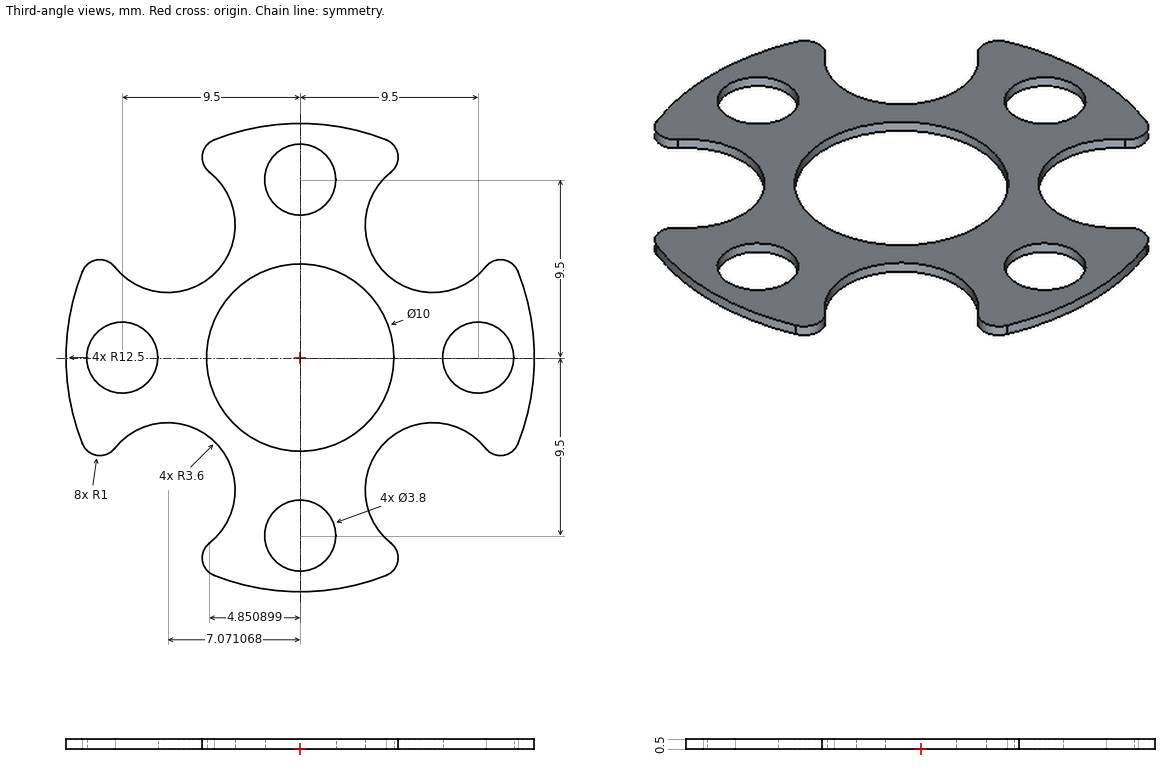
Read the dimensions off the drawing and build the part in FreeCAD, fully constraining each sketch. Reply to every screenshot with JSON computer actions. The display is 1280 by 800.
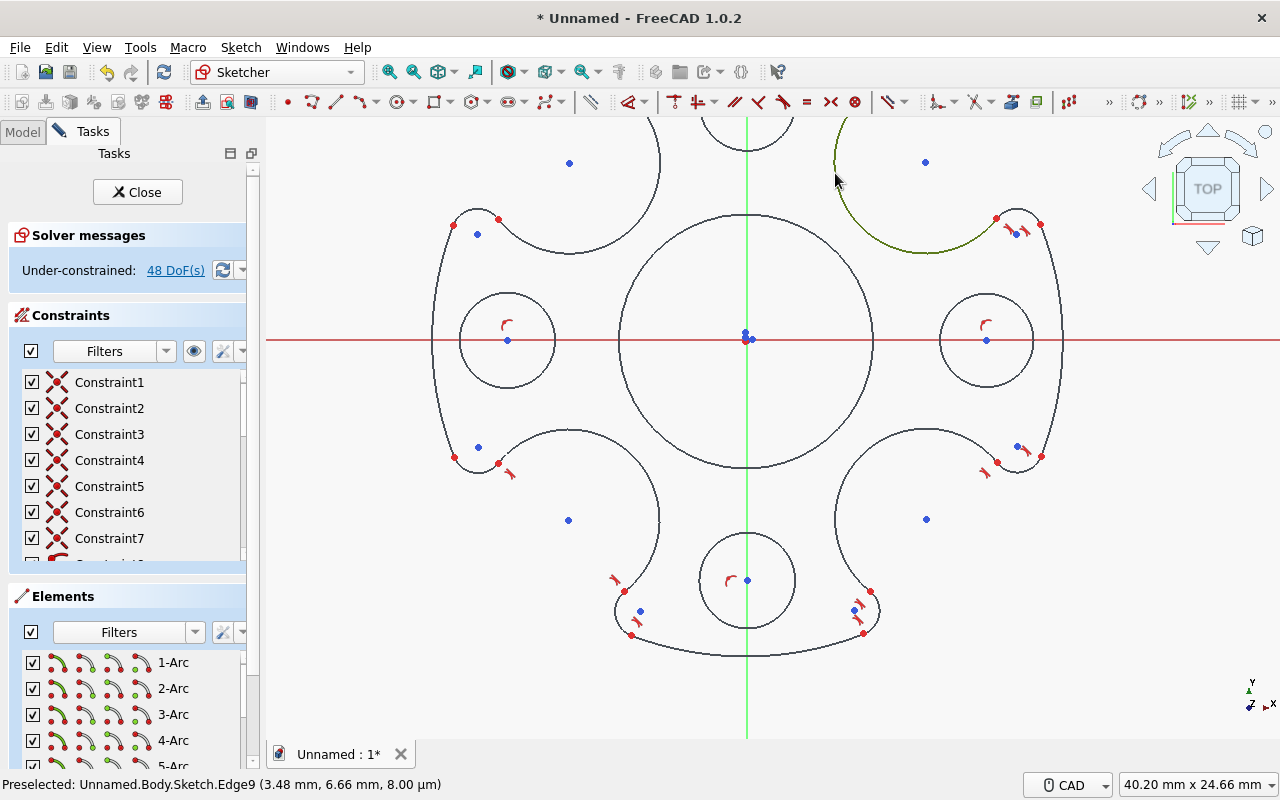
{"action": "scroll", "coordinate": [618, 606], "scroll_direction": "down", "scroll_amount": 2}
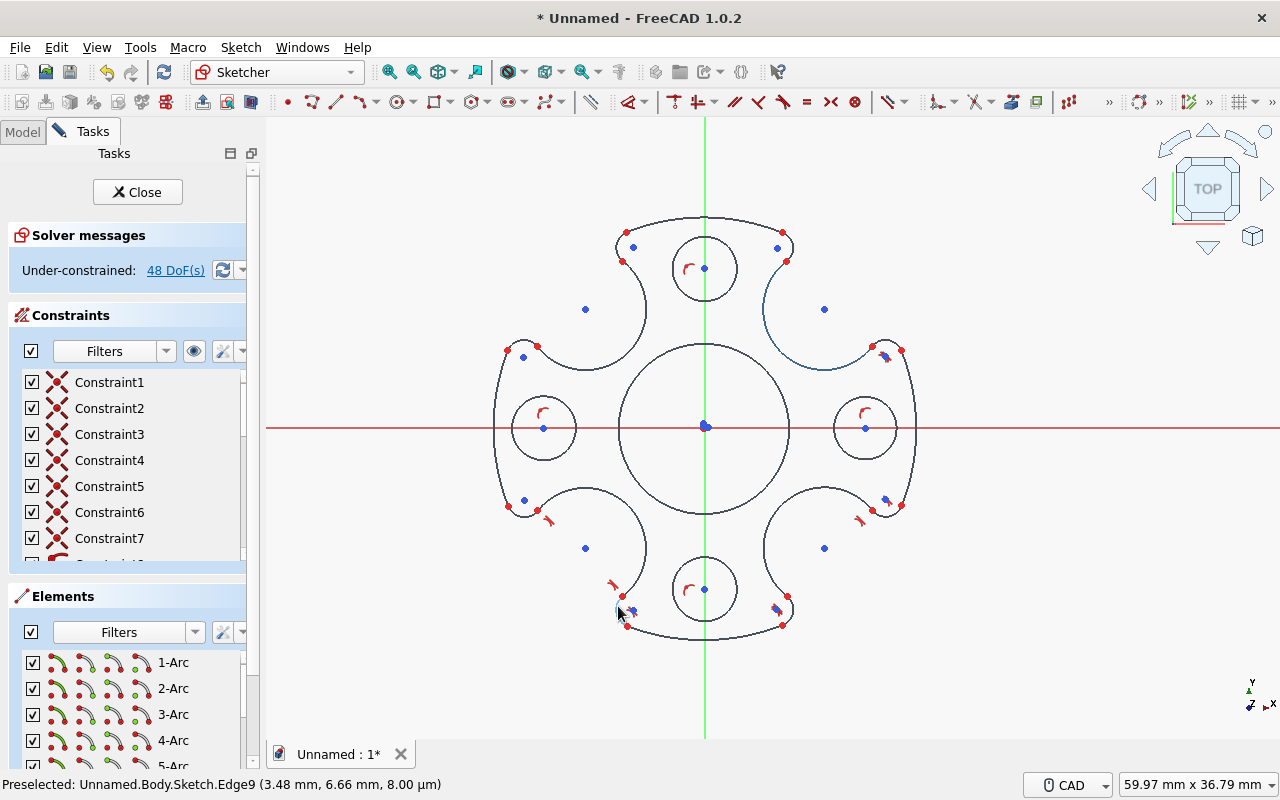
{"action": "scroll", "coordinate": [793, 253], "scroll_direction": "up", "scroll_amount": 2}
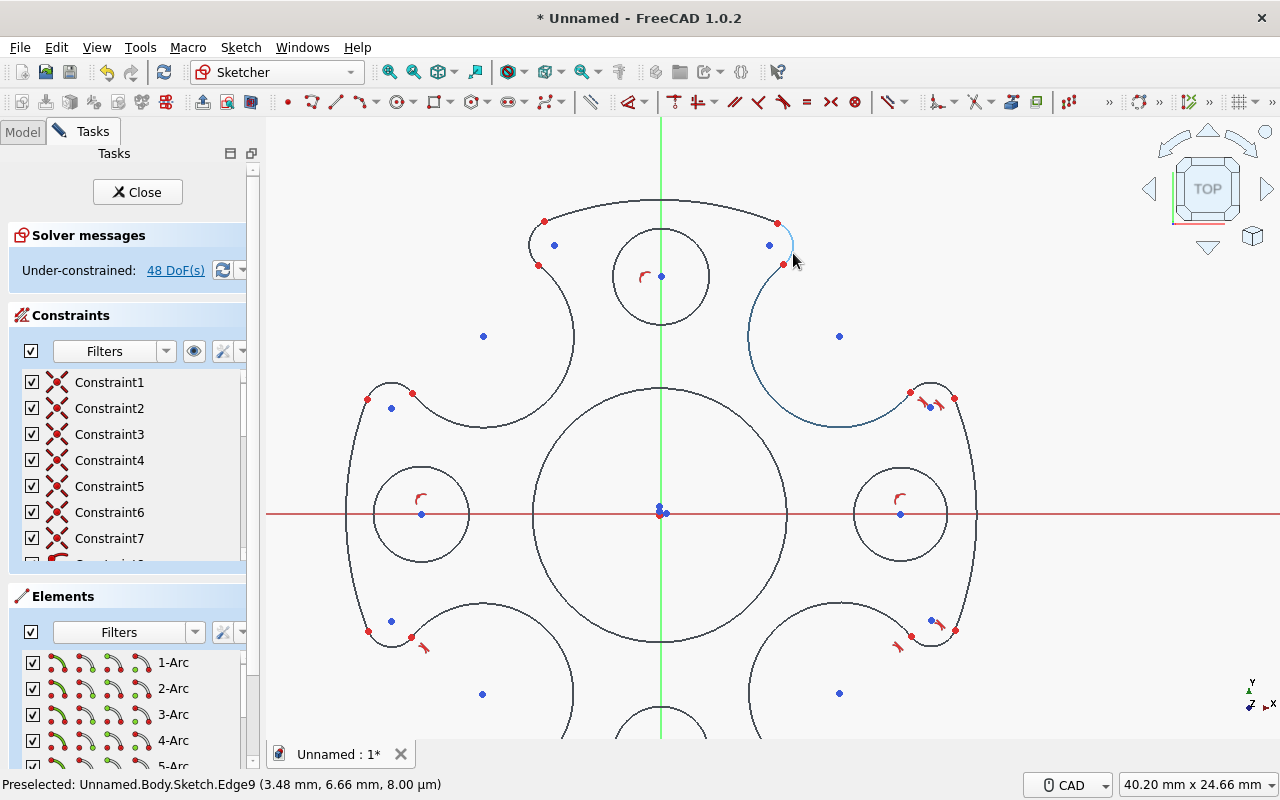
{"action": "left_click", "coordinate": [792, 253]}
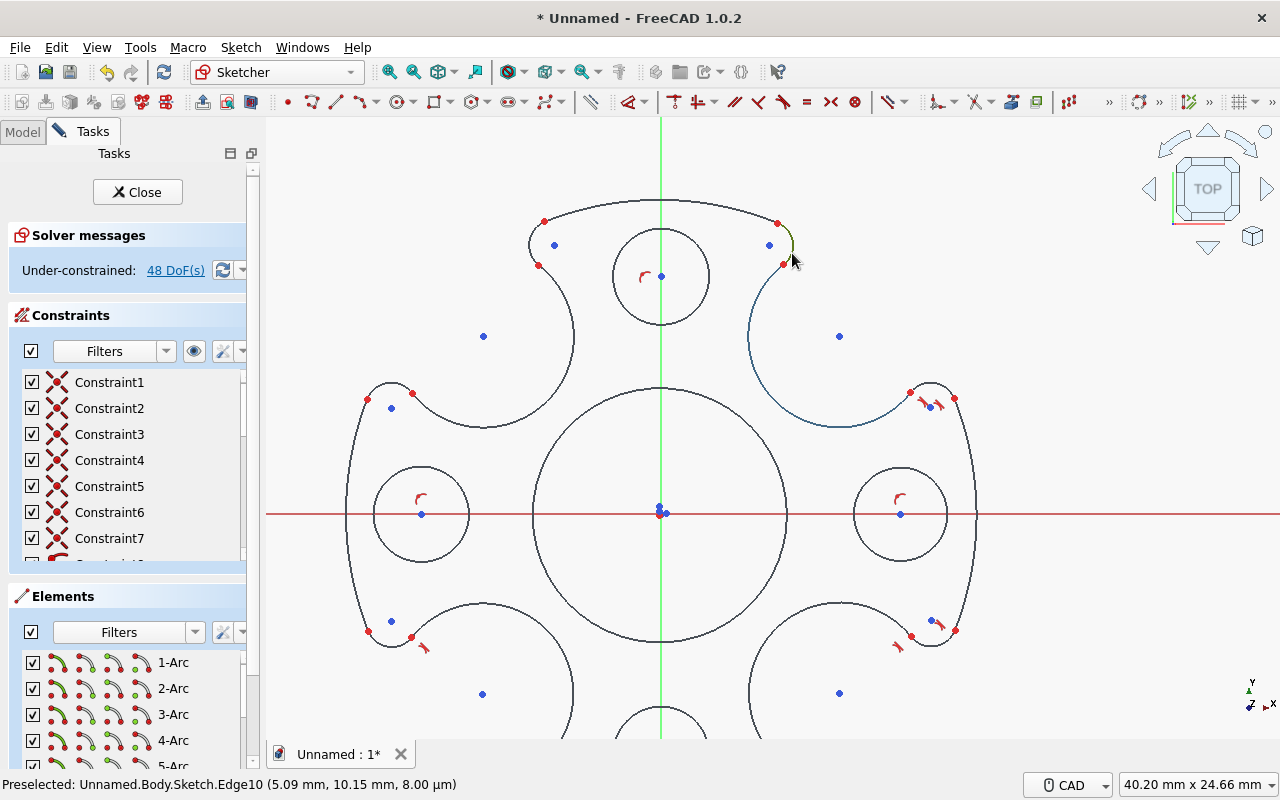
{"action": "key", "text": "t"}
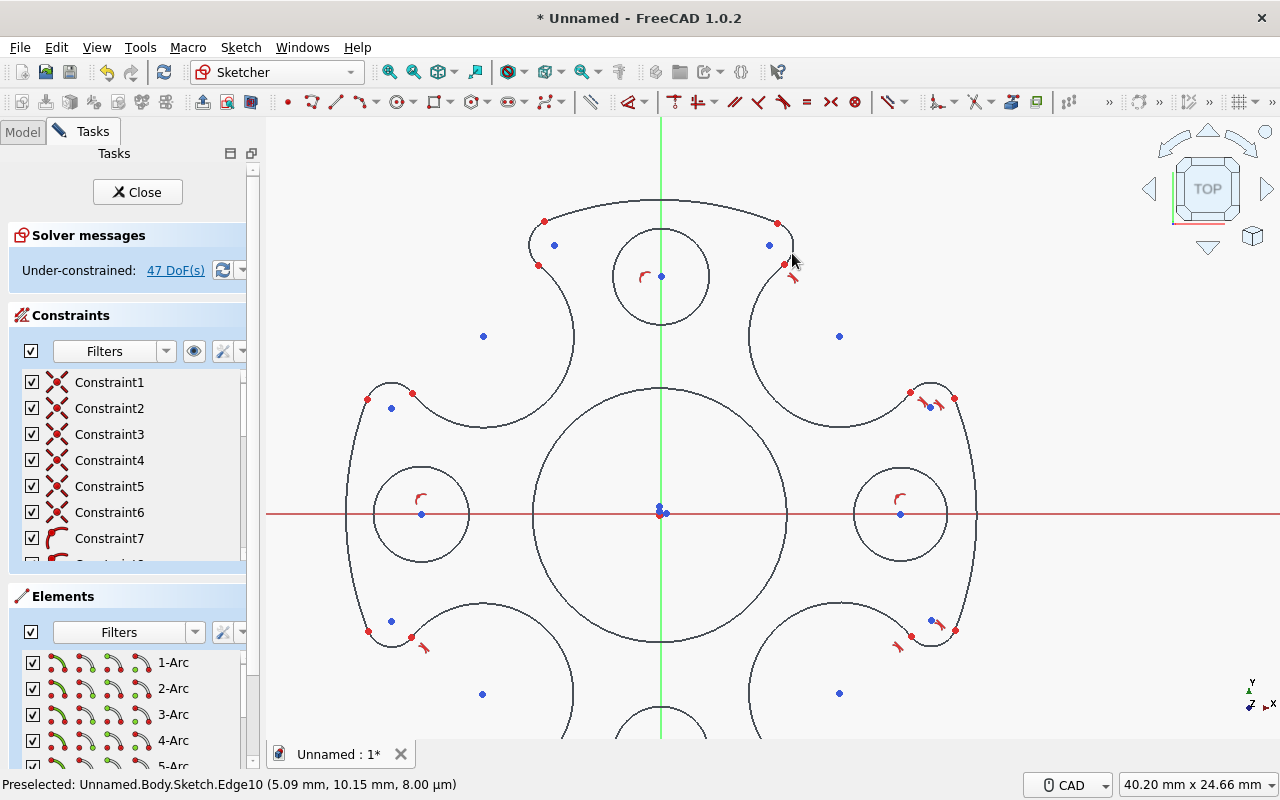
{"action": "left_click", "coordinate": [793, 252]}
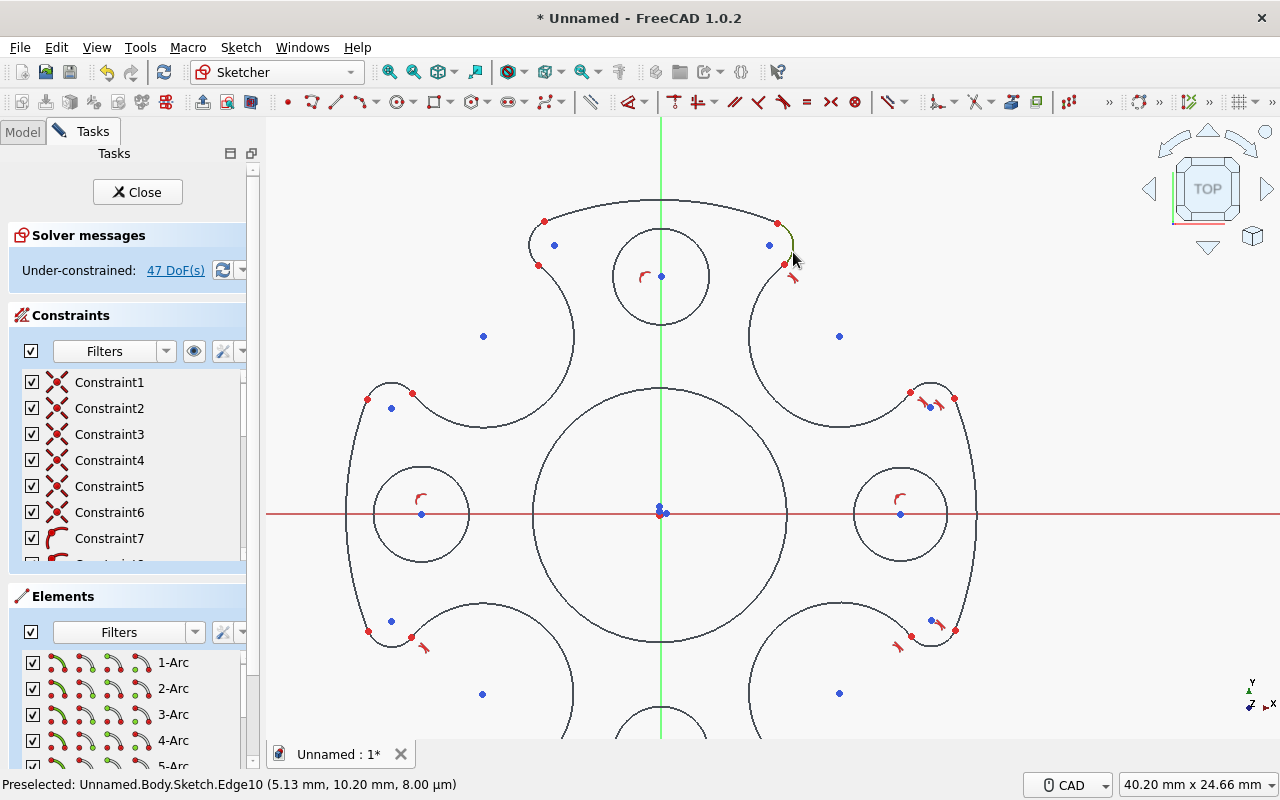
{"action": "left_click", "coordinate": [709, 204]}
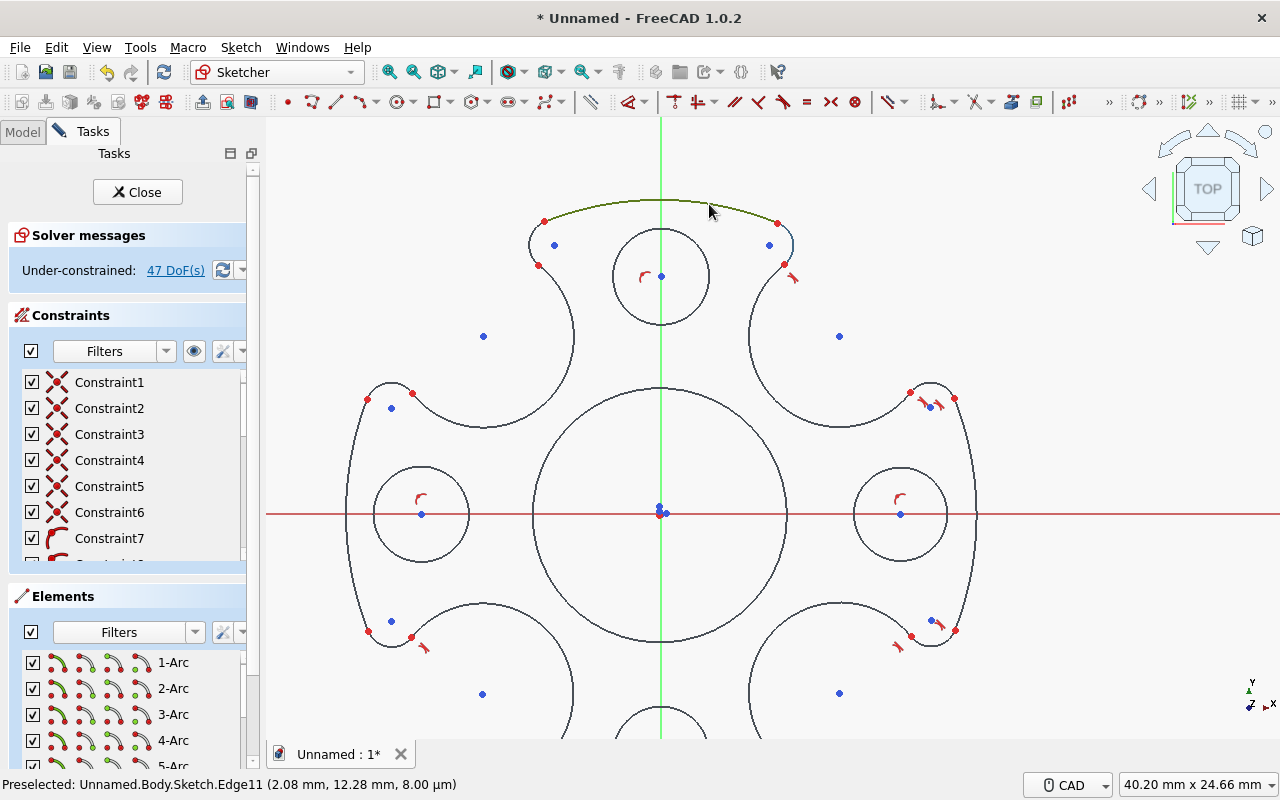
{"action": "left_click", "coordinate": [784, 102]}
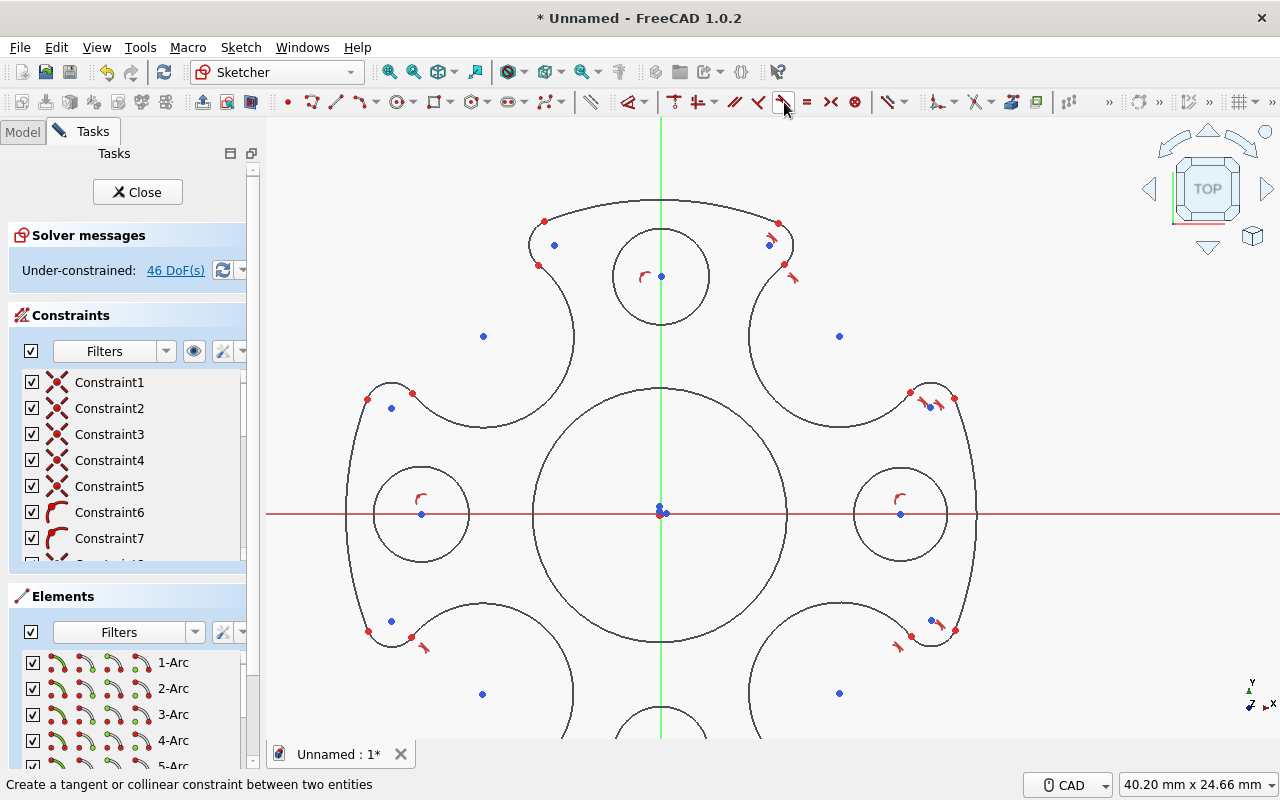
{"action": "left_click", "coordinate": [709, 204]}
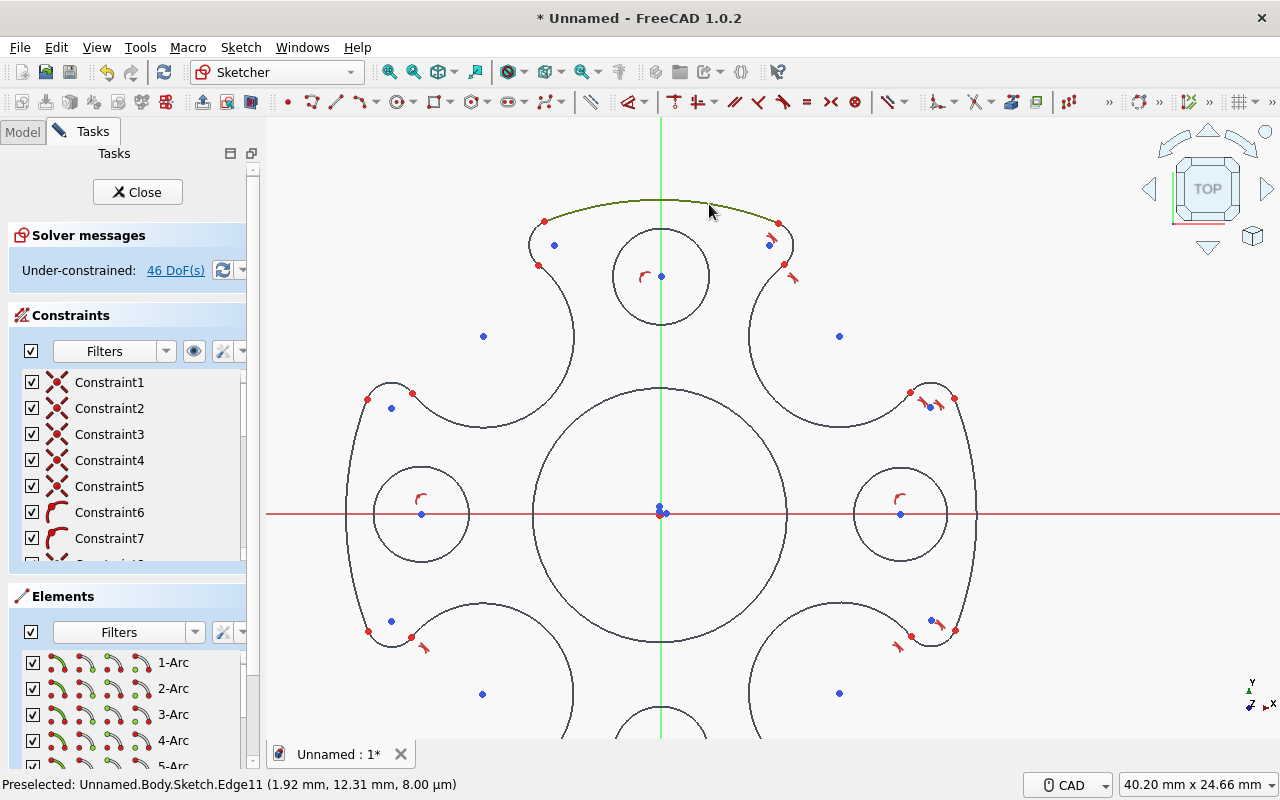
{"action": "left_click", "coordinate": [533, 232]}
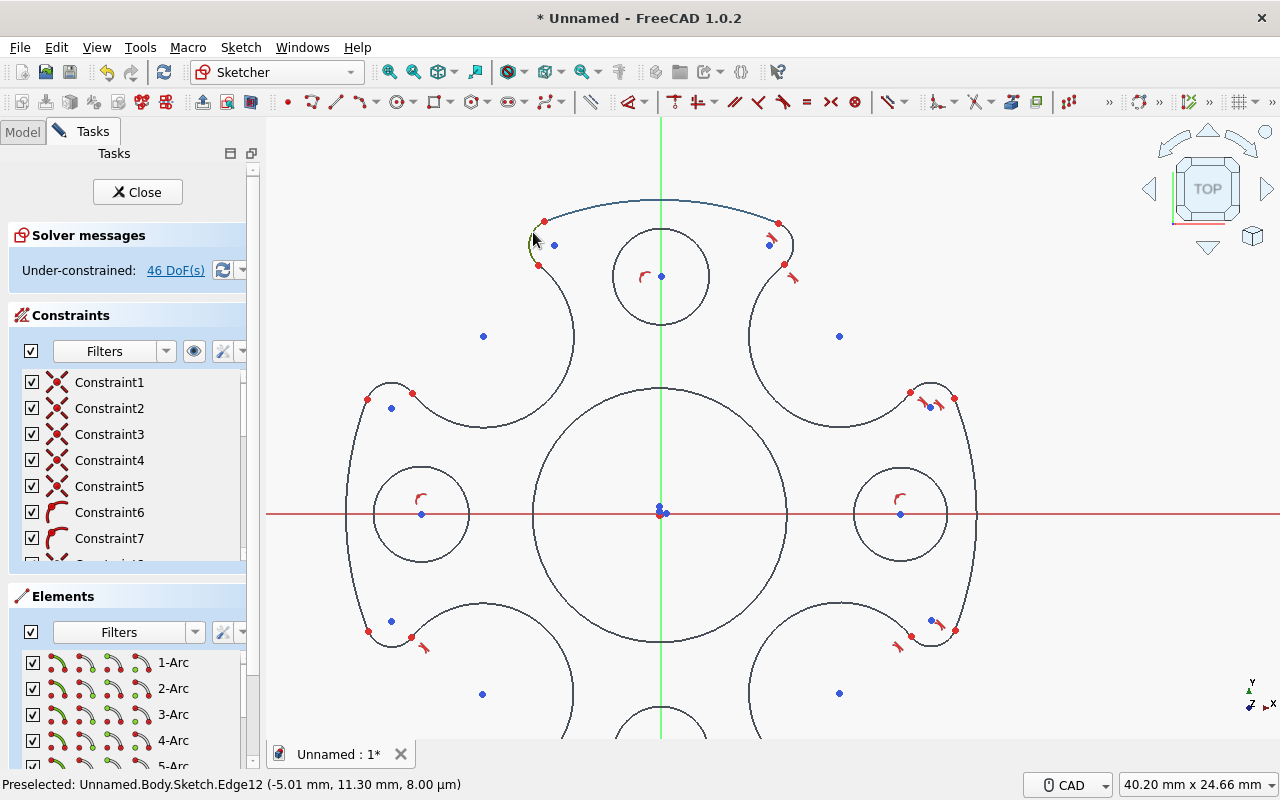
{"action": "left_click", "coordinate": [784, 102]}